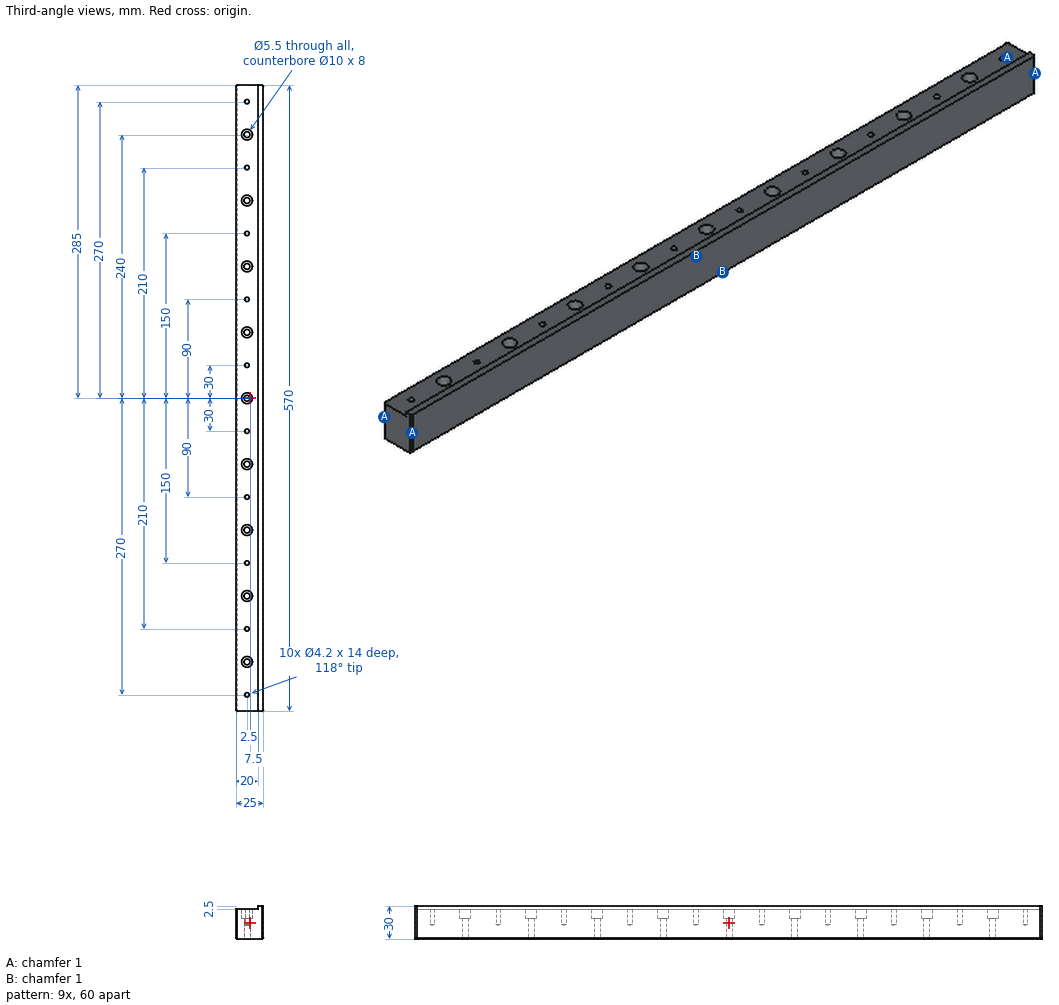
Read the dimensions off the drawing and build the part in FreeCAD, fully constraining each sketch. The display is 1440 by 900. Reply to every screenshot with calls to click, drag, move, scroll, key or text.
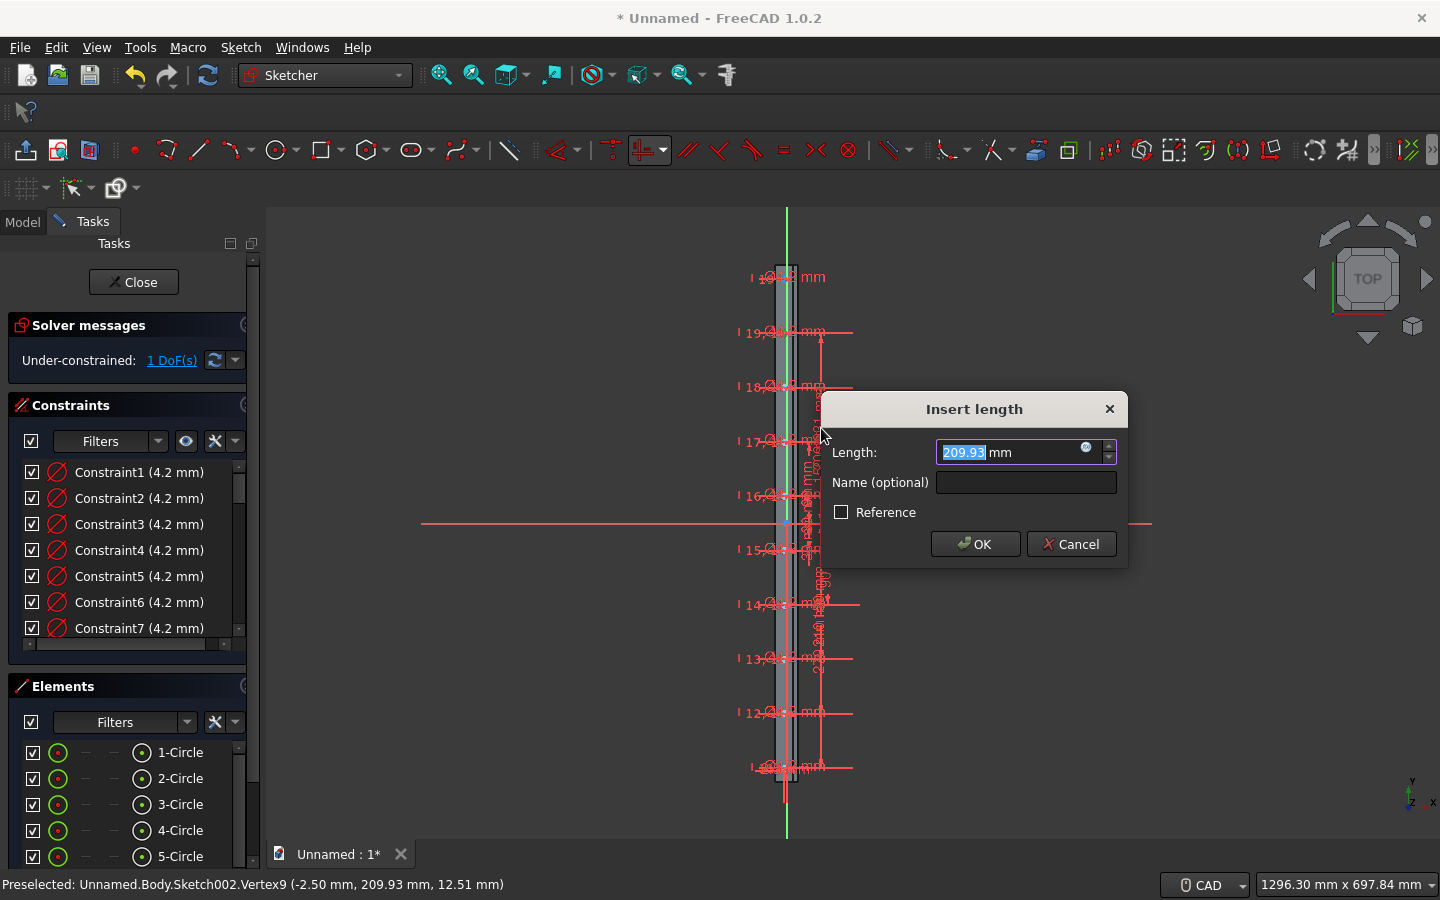
text(210)
key(Return)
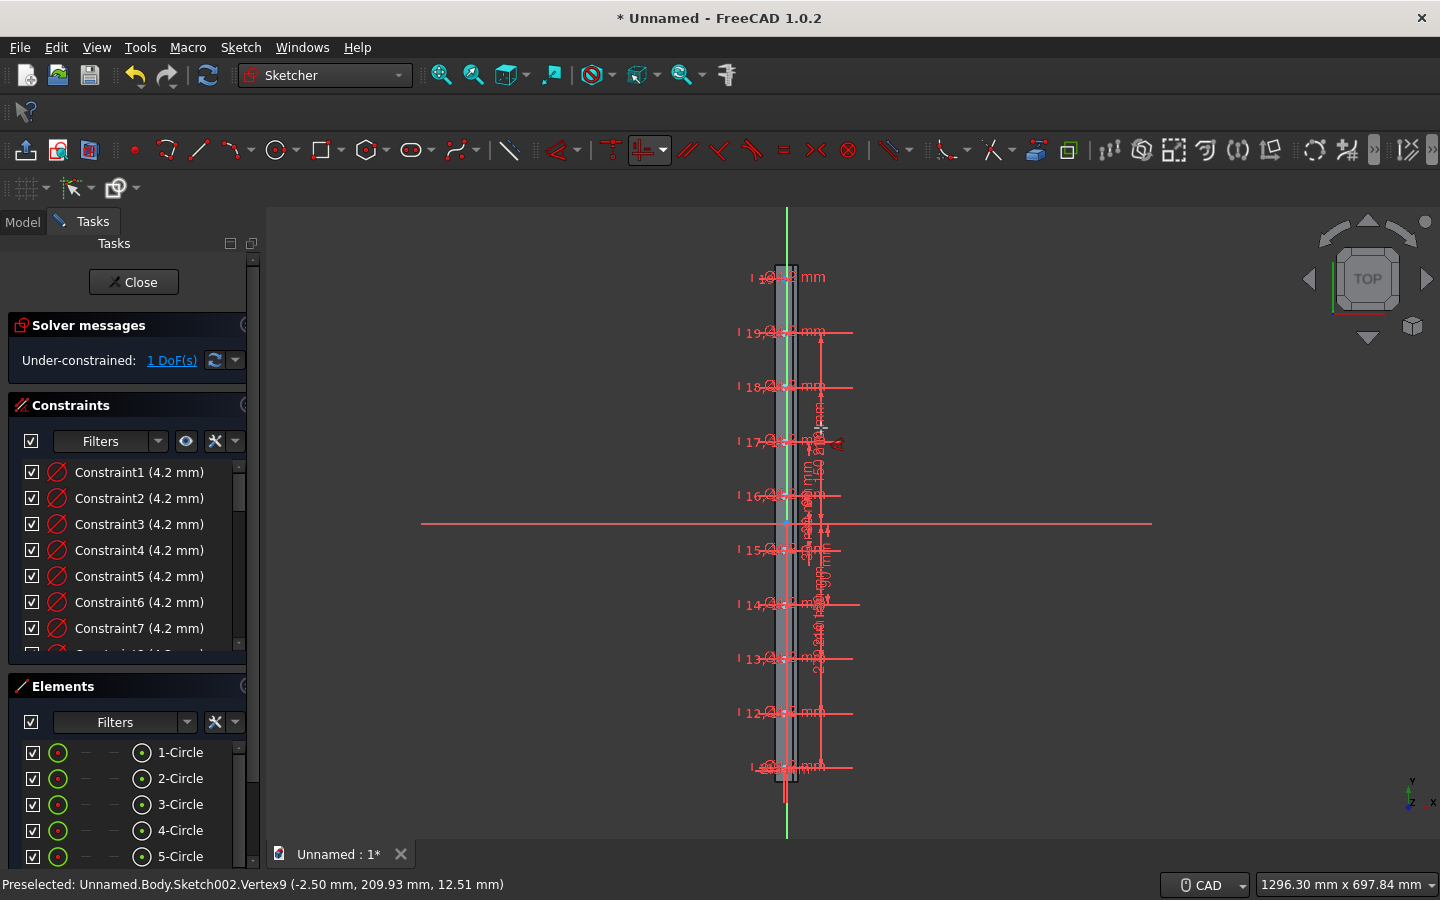
click(784, 279)
click(821, 401)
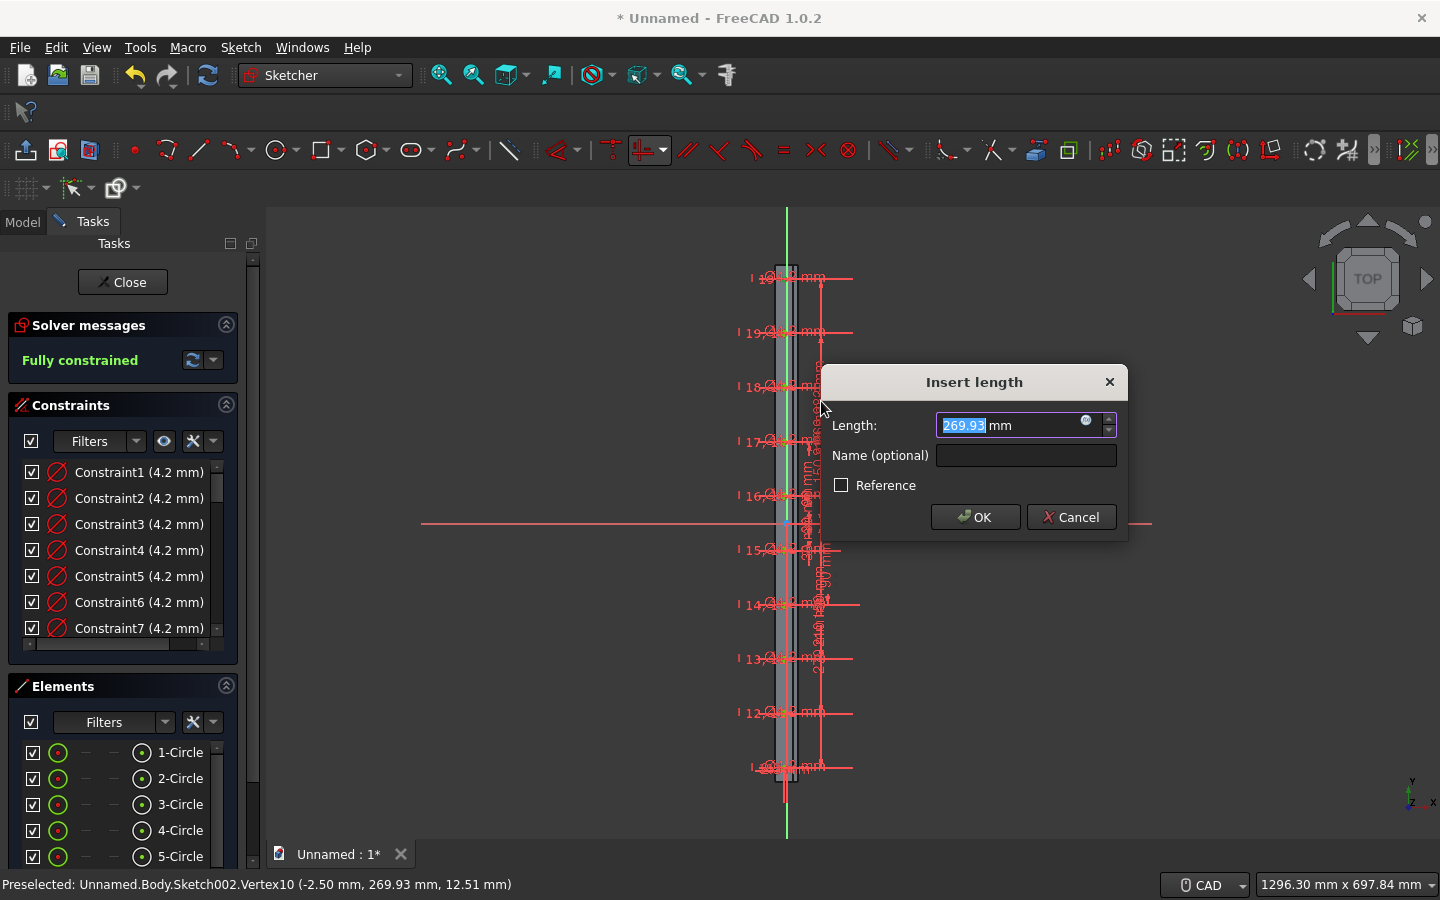
text(270)
key(Return)
key(Escape)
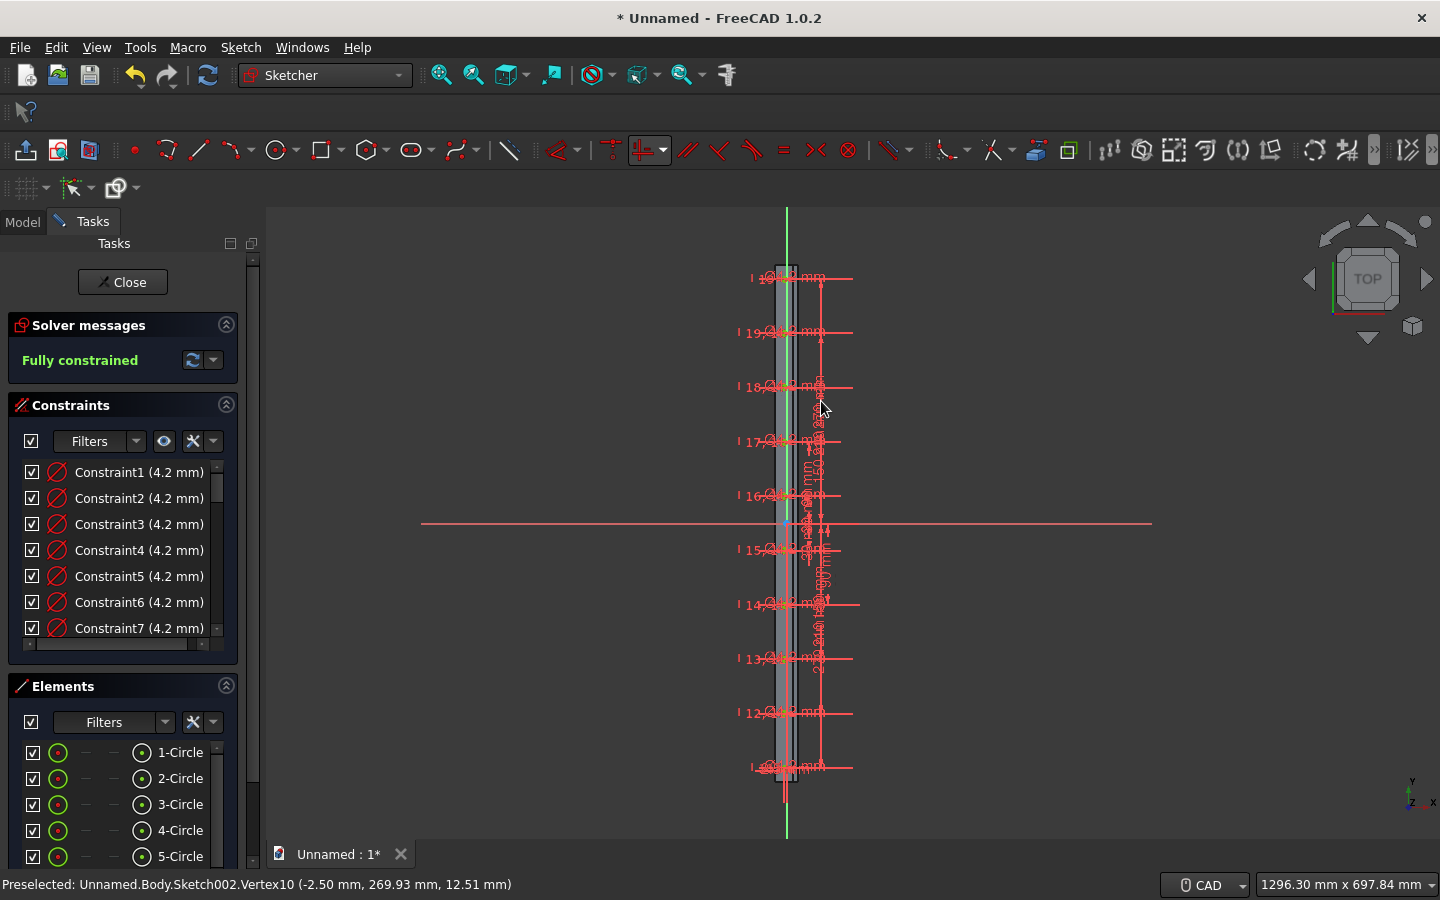
click(123, 282)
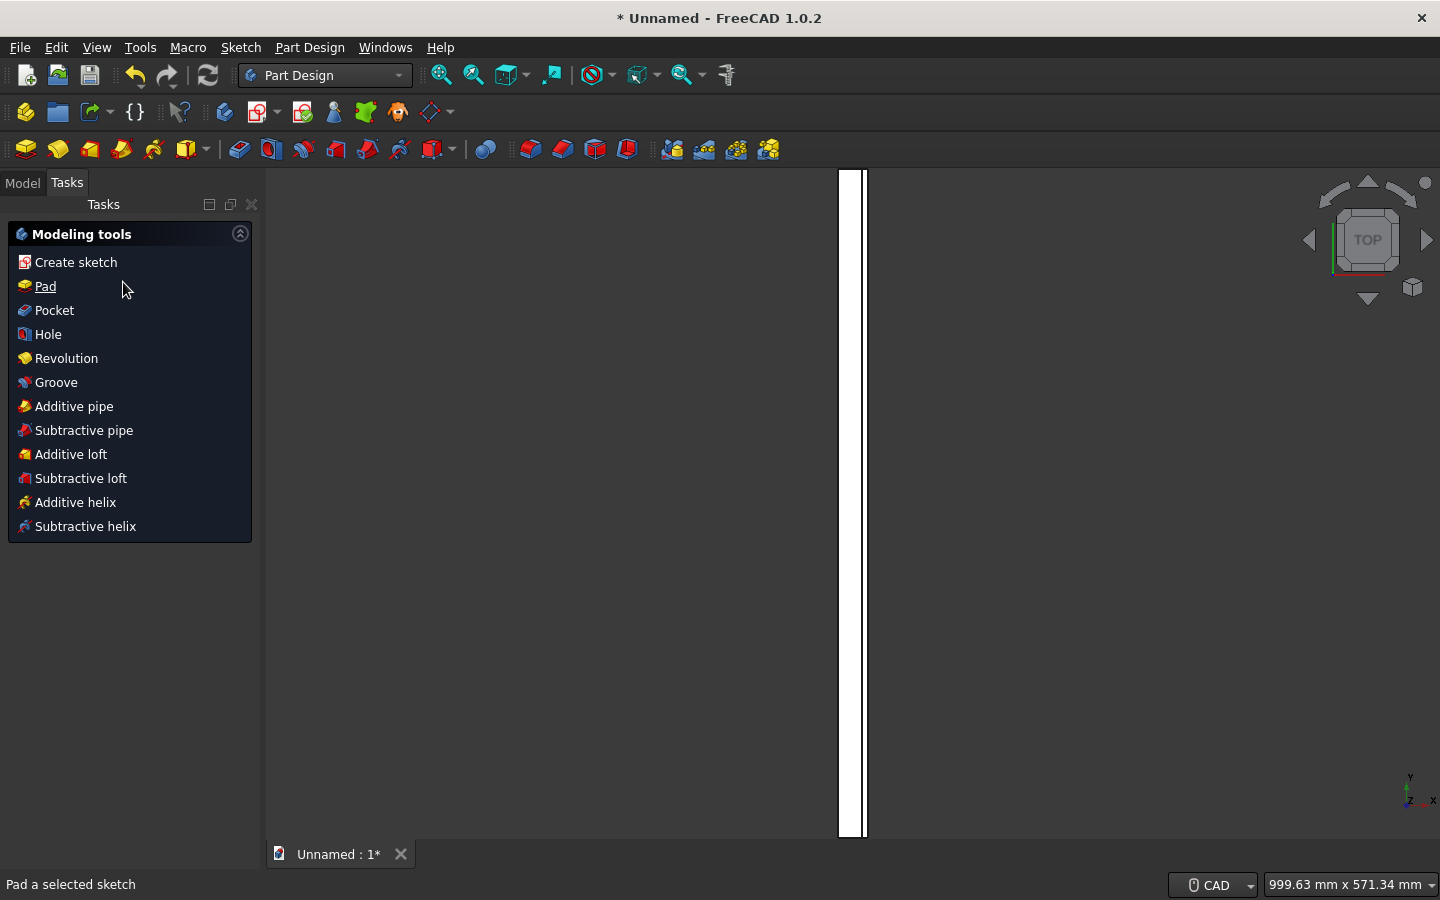
click(272, 150)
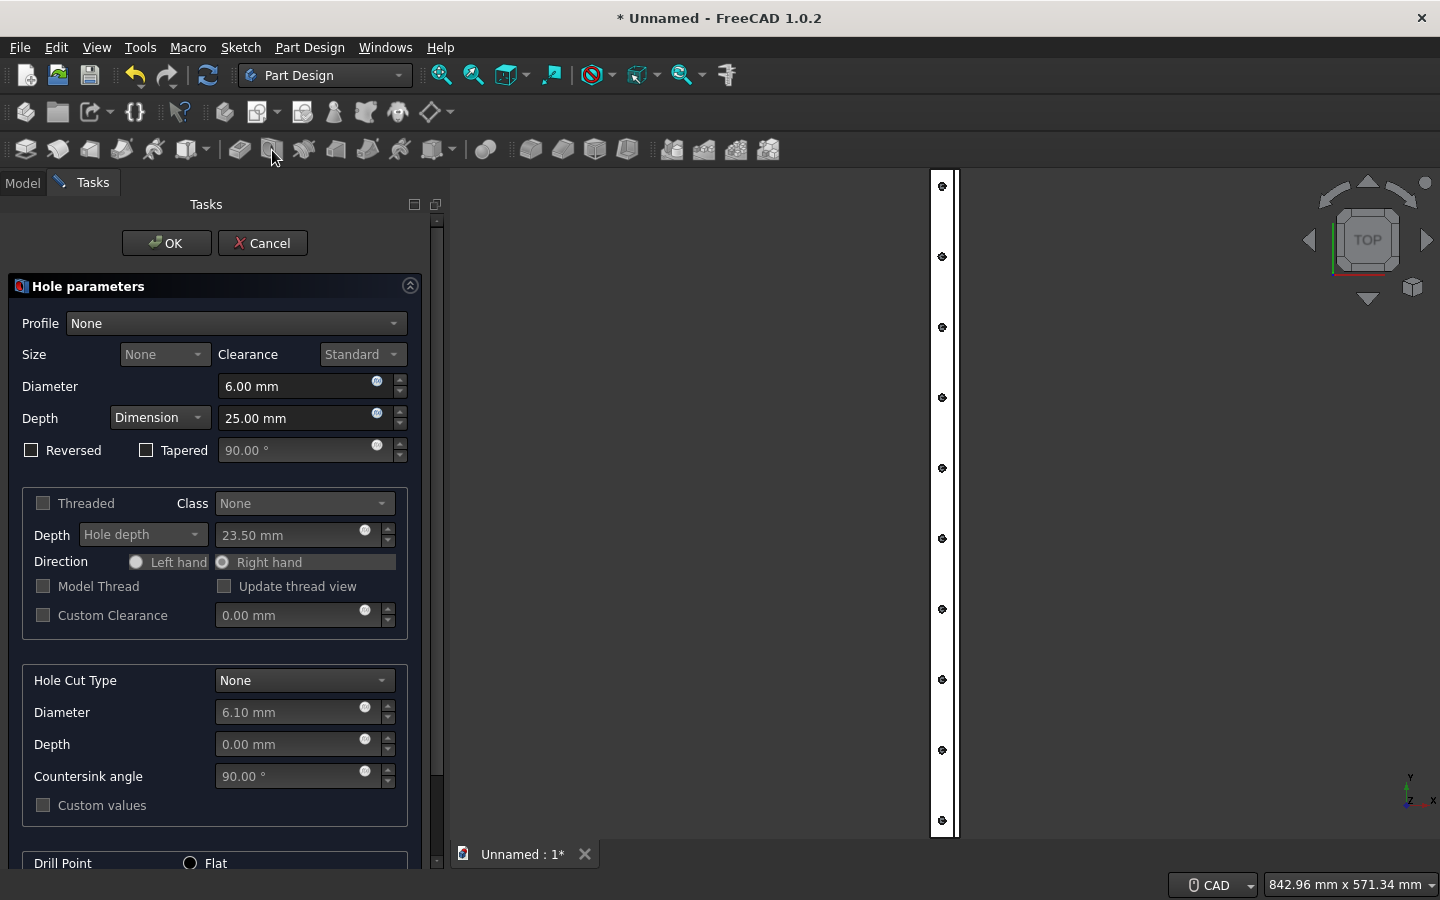
triple_click(305, 386)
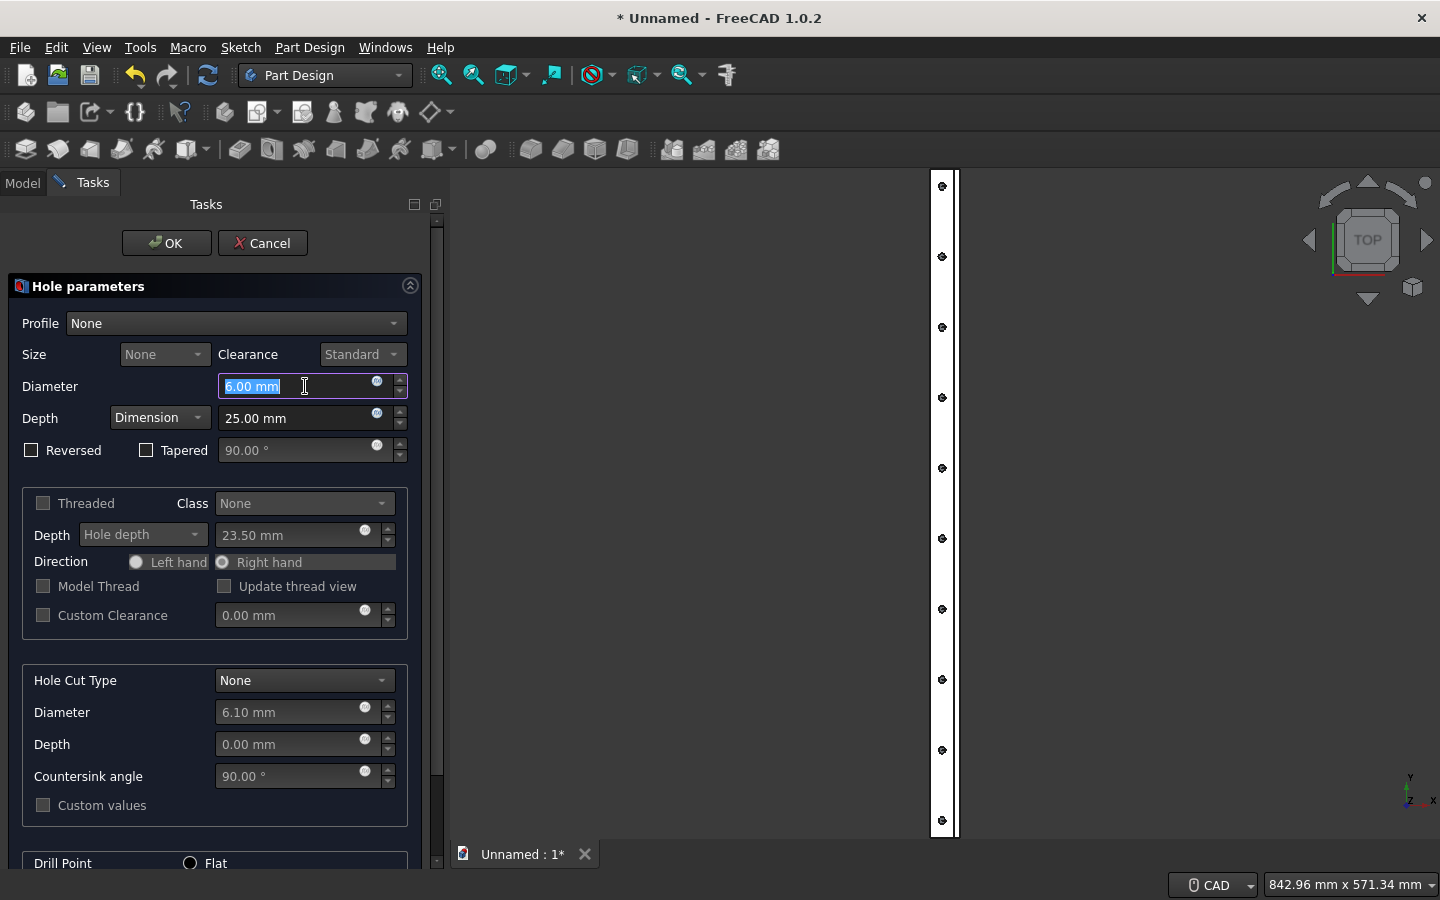
text(4.2)
key(Tab)